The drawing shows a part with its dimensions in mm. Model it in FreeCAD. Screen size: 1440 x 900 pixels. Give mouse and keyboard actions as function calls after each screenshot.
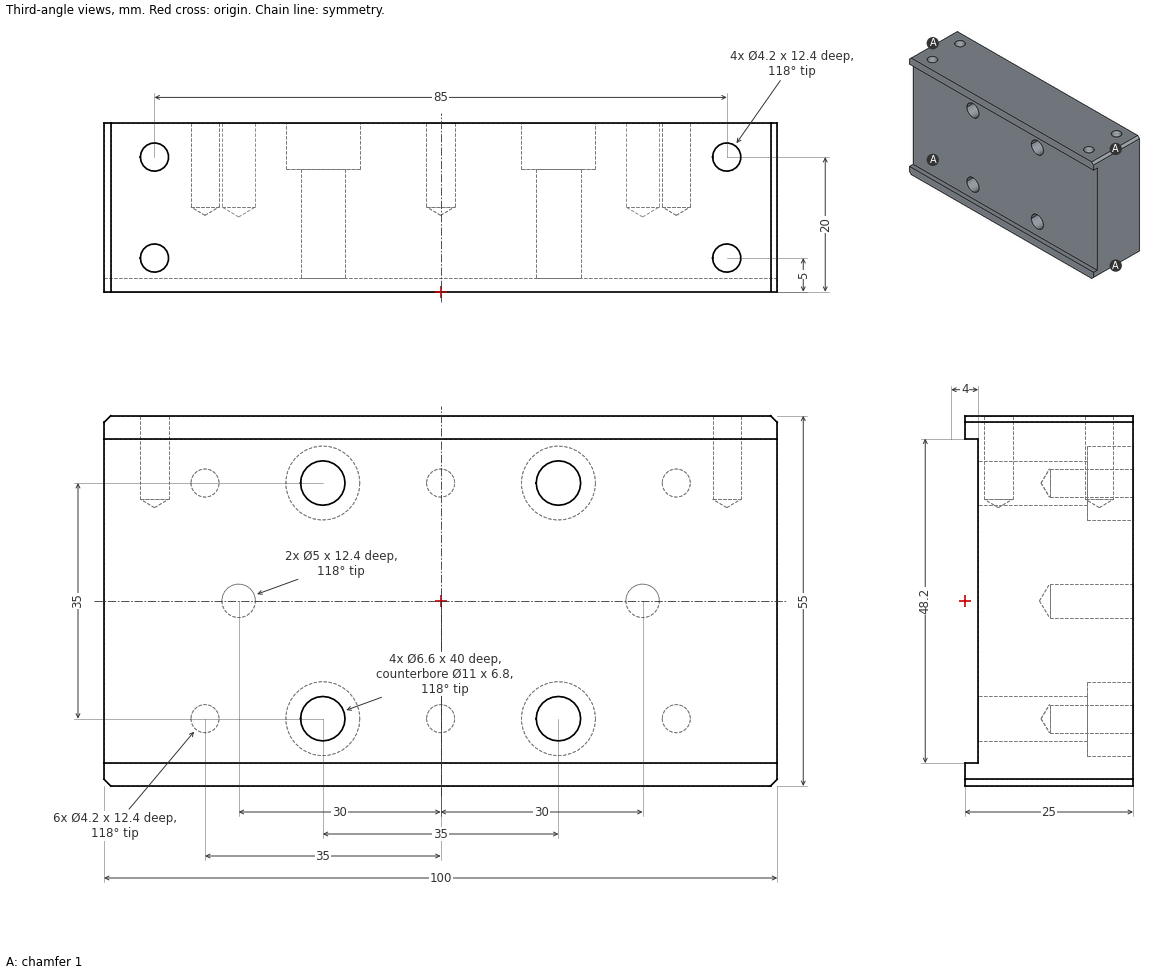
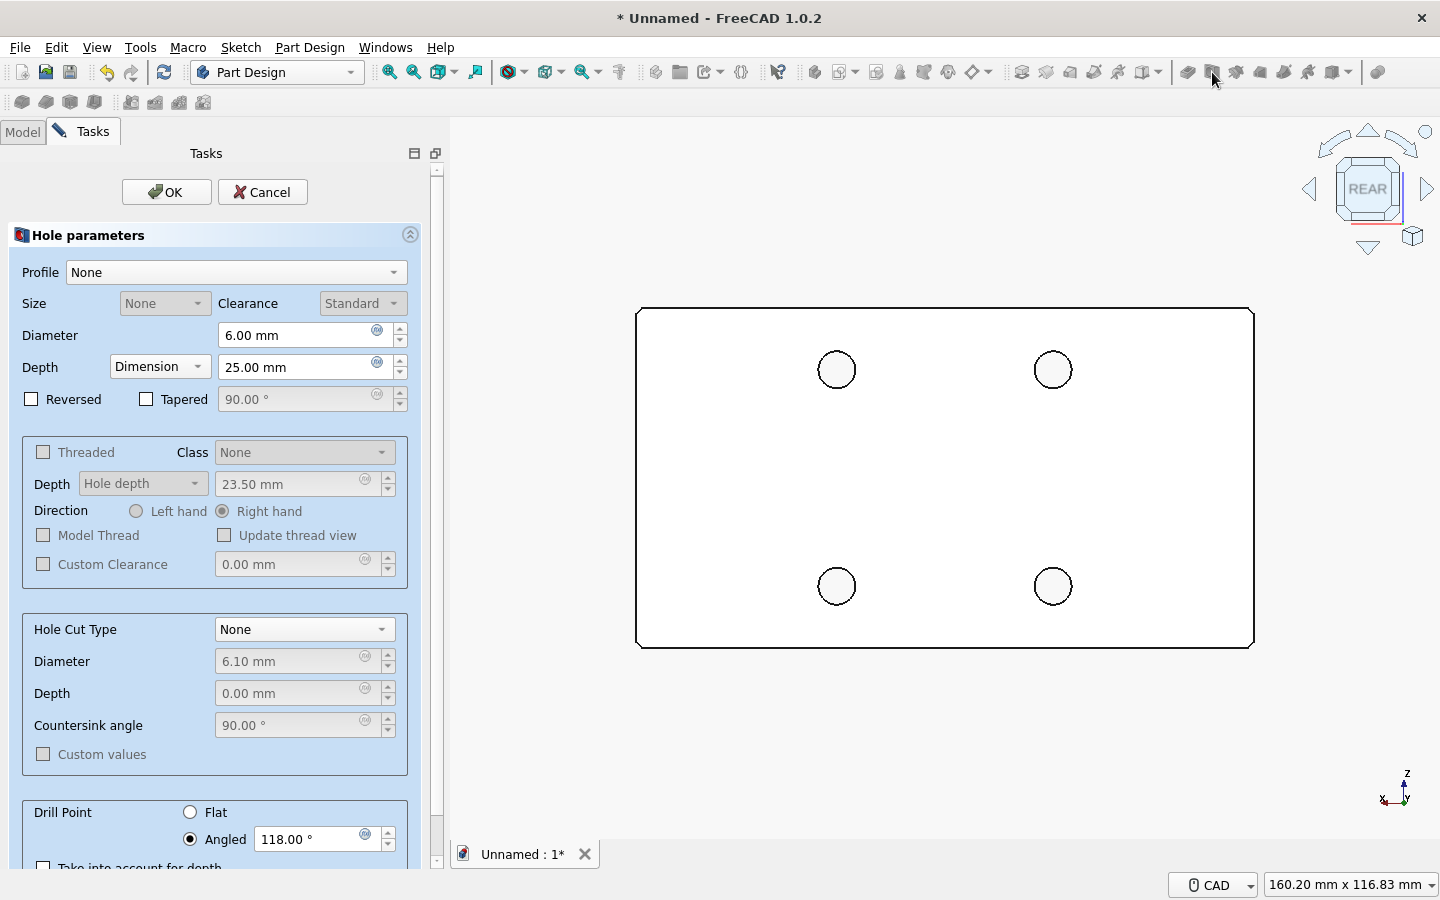
triple_click(305, 335)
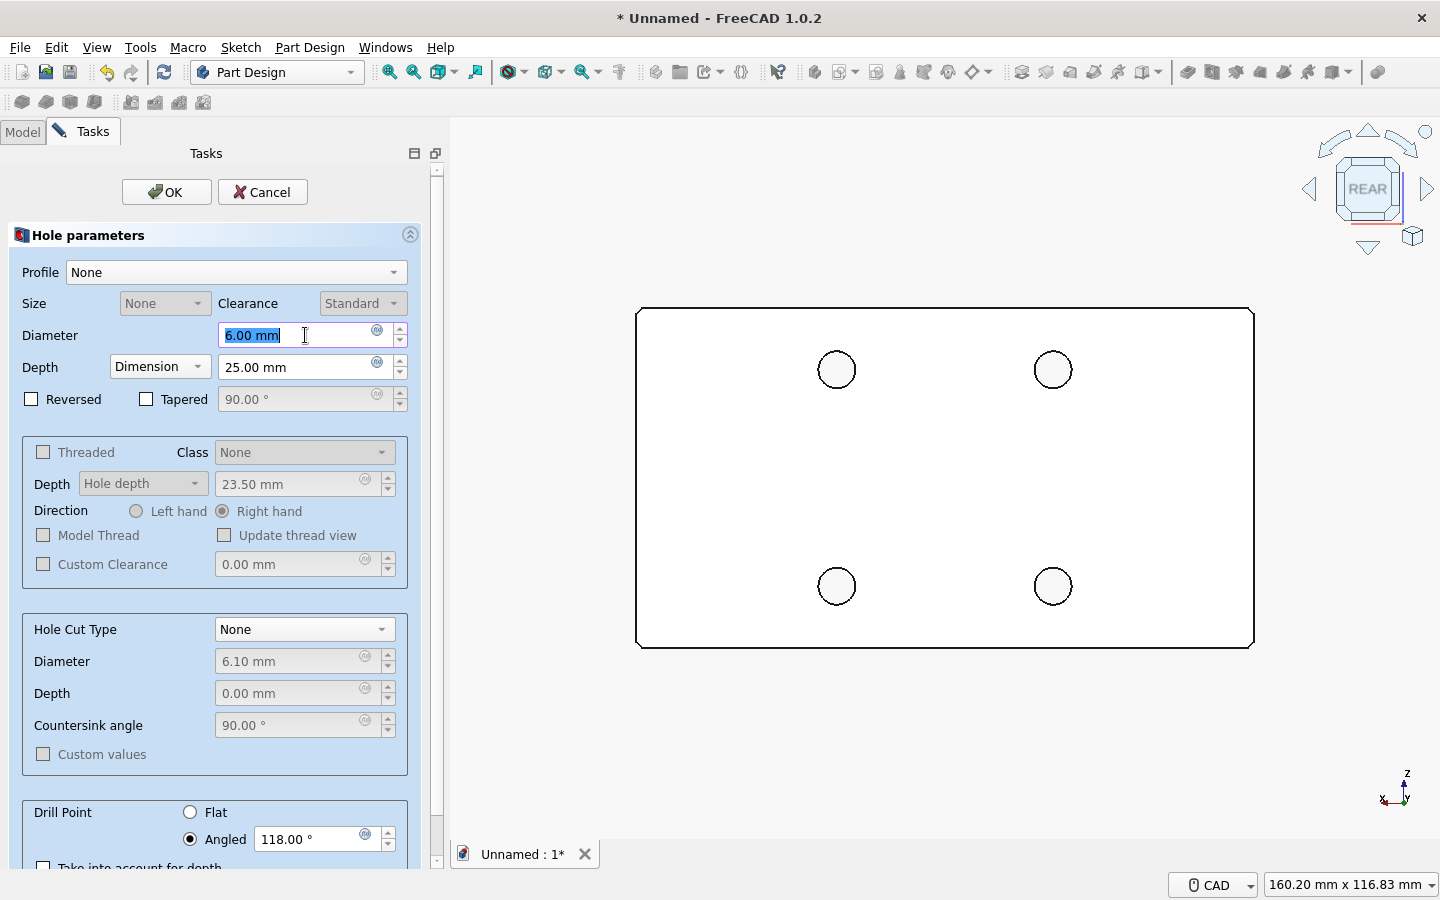
text(6.6)
key(Tab)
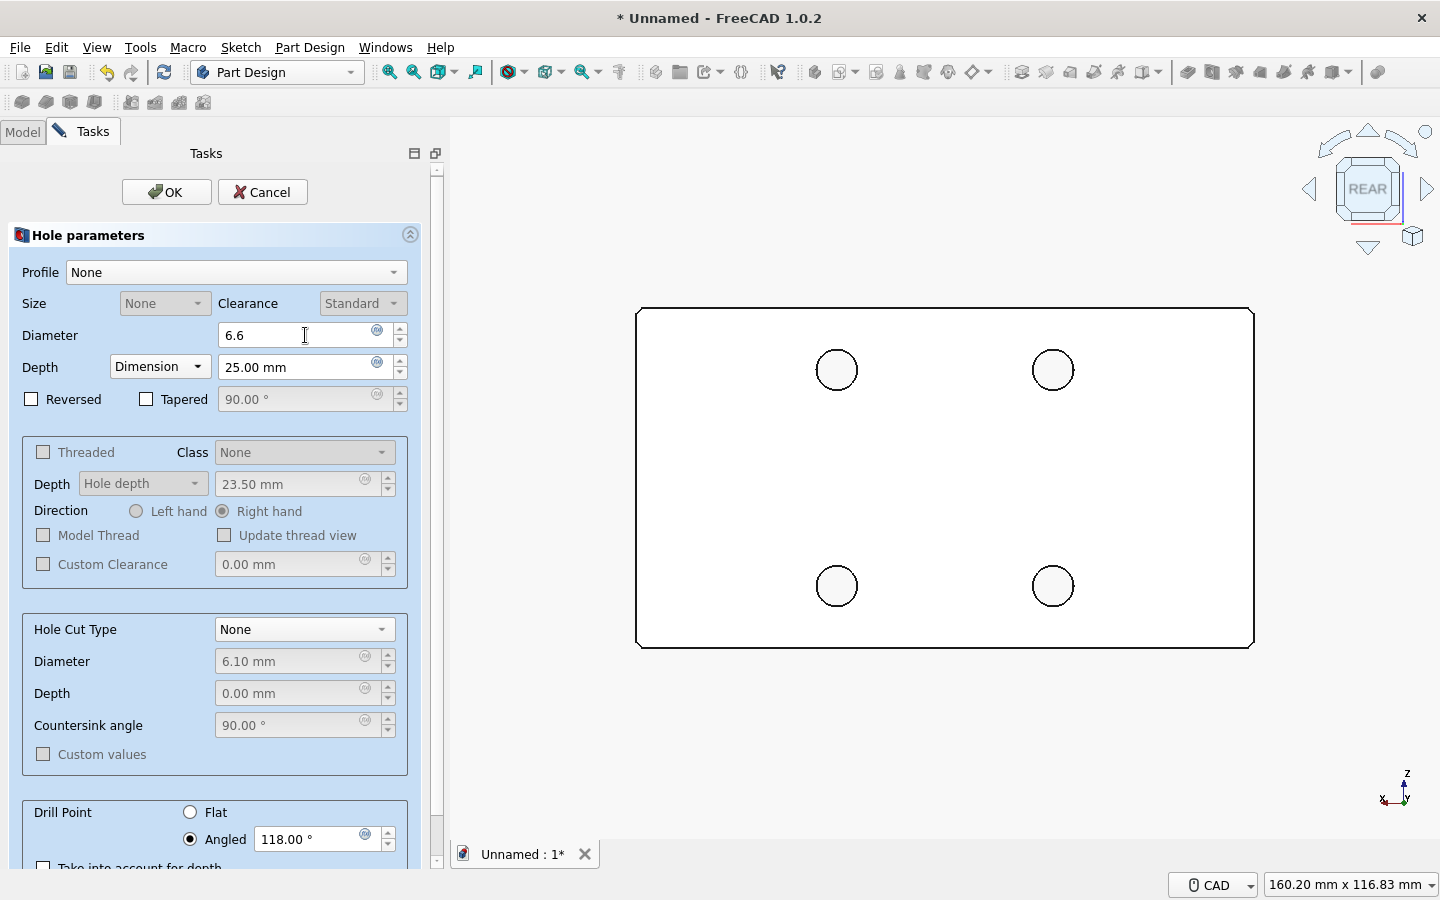
triple_click(305, 367)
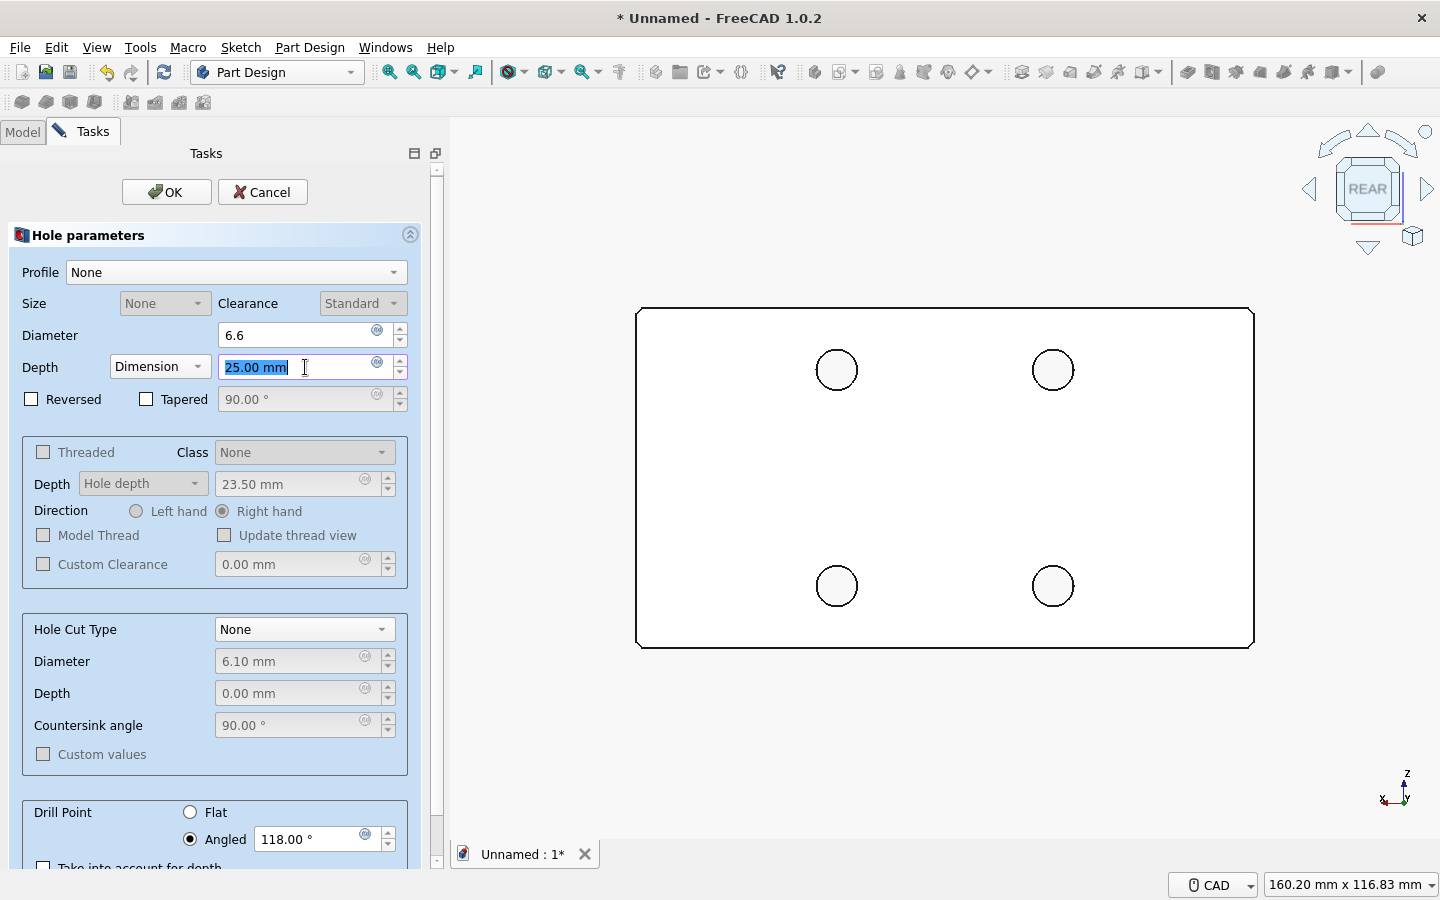
text(40)
key(Tab)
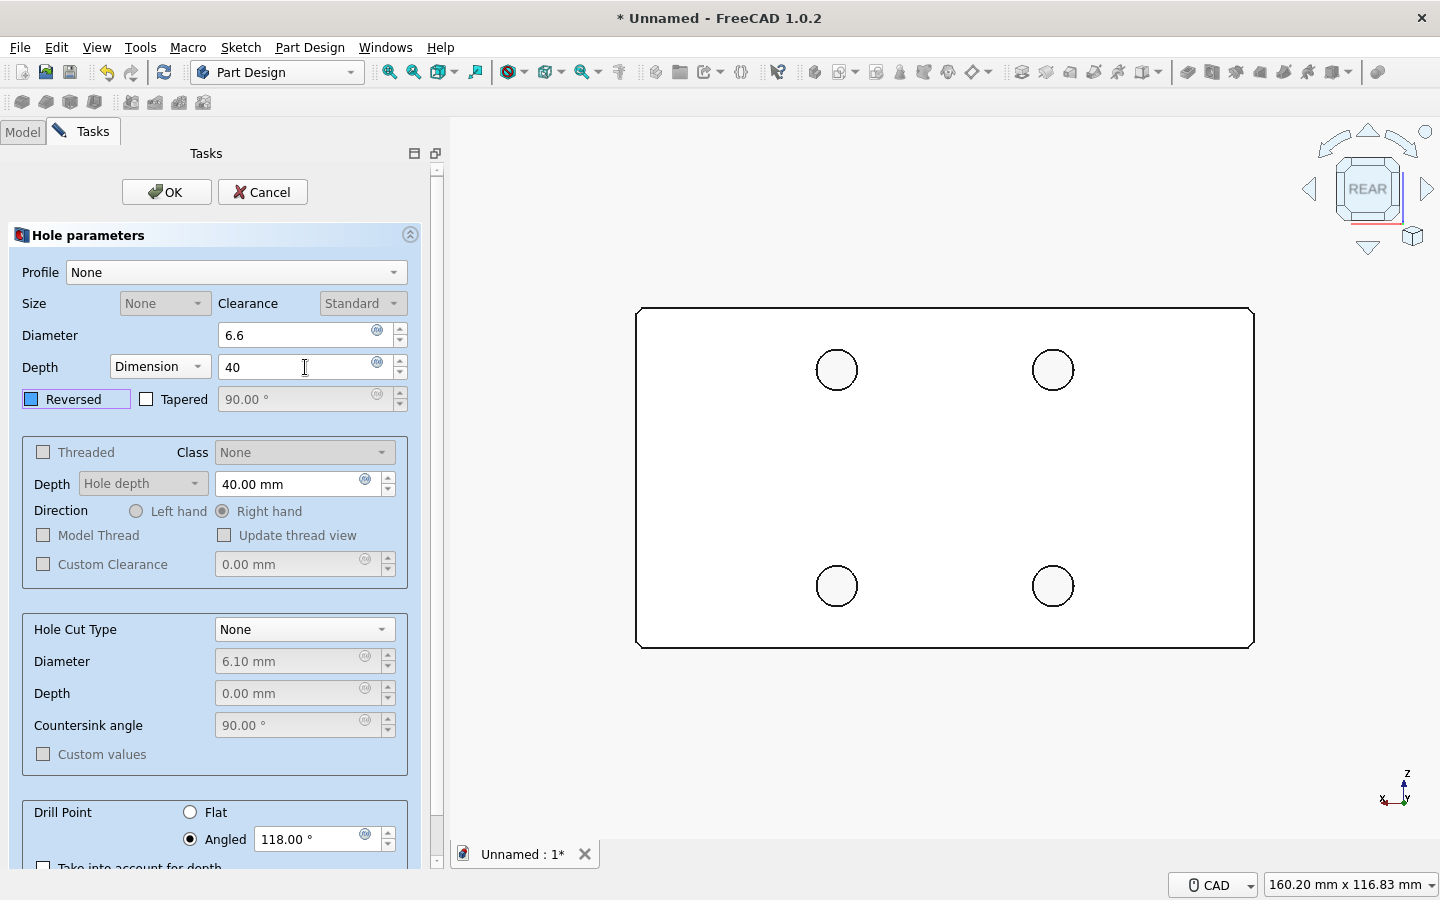
click(306, 630)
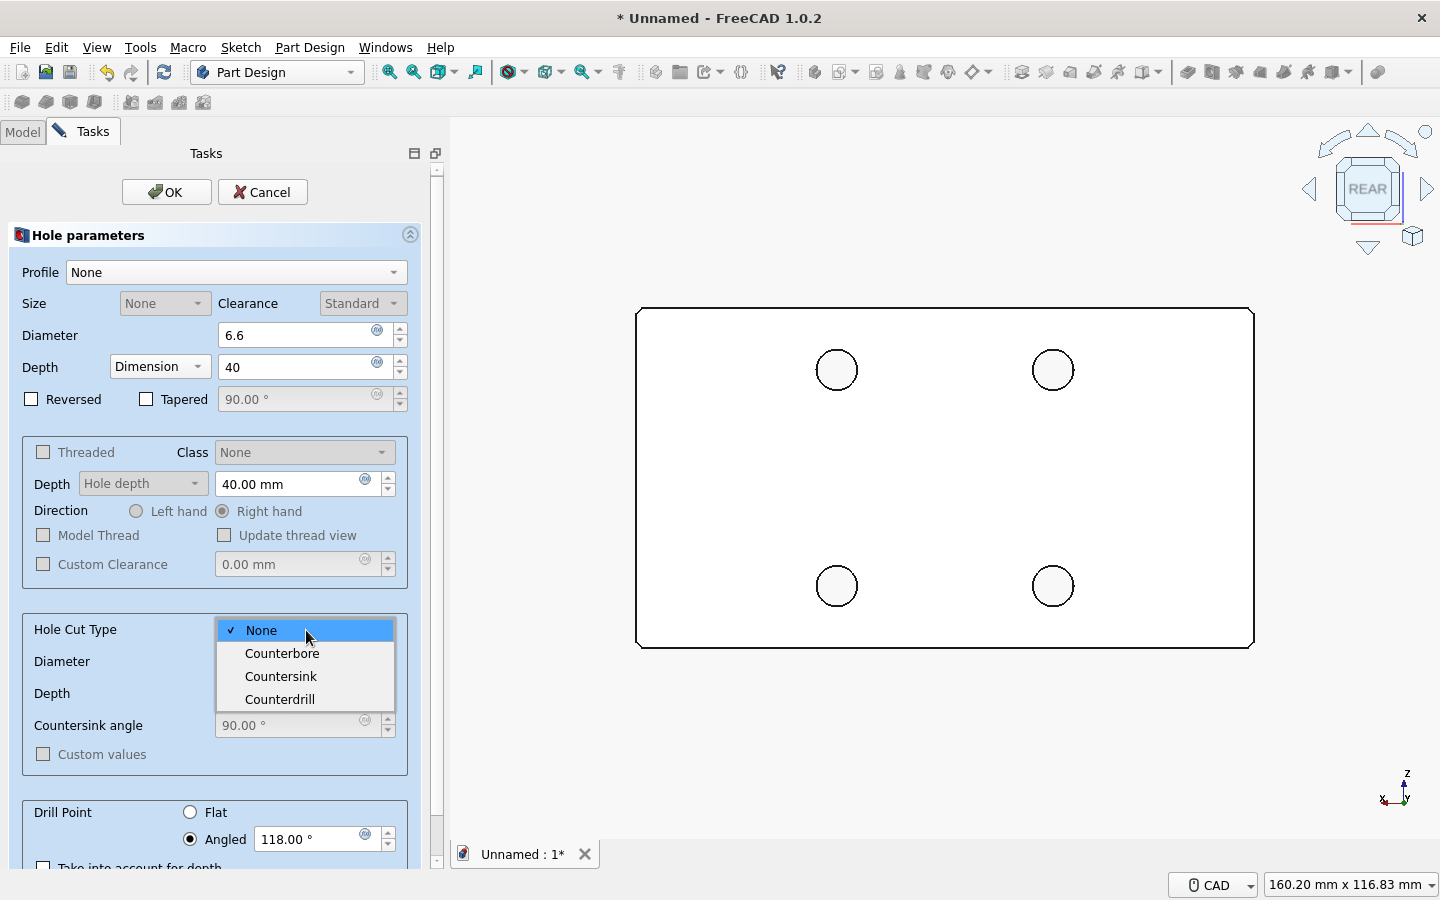
click(304, 654)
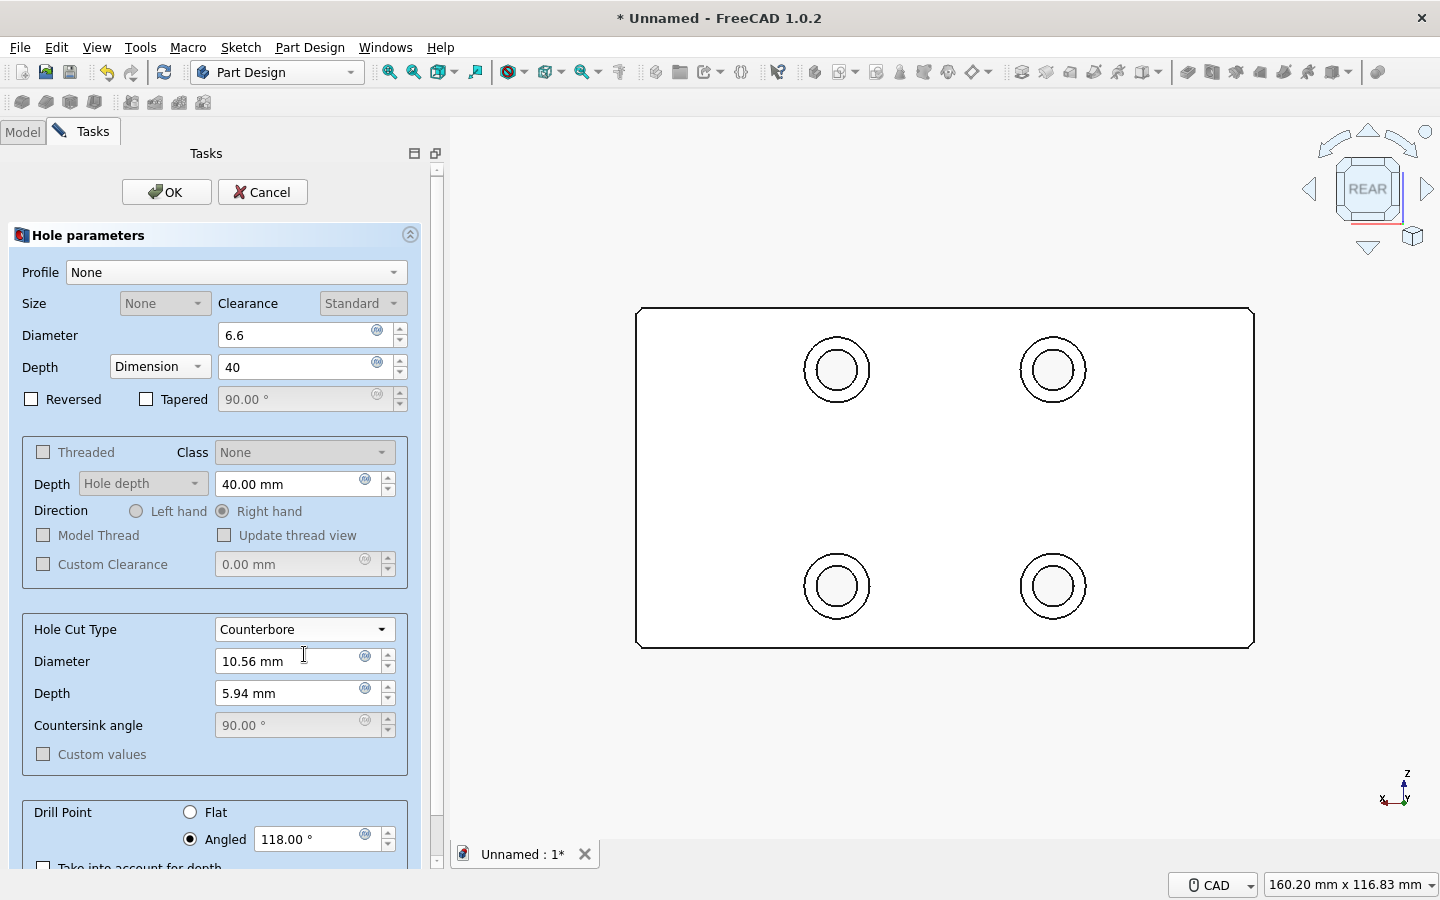
triple_click(298, 661)